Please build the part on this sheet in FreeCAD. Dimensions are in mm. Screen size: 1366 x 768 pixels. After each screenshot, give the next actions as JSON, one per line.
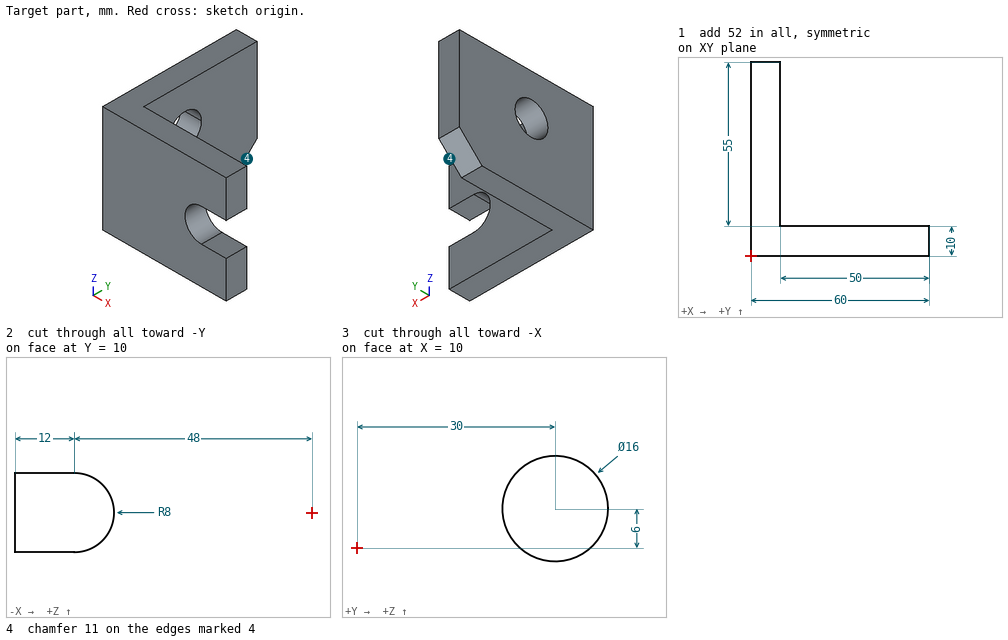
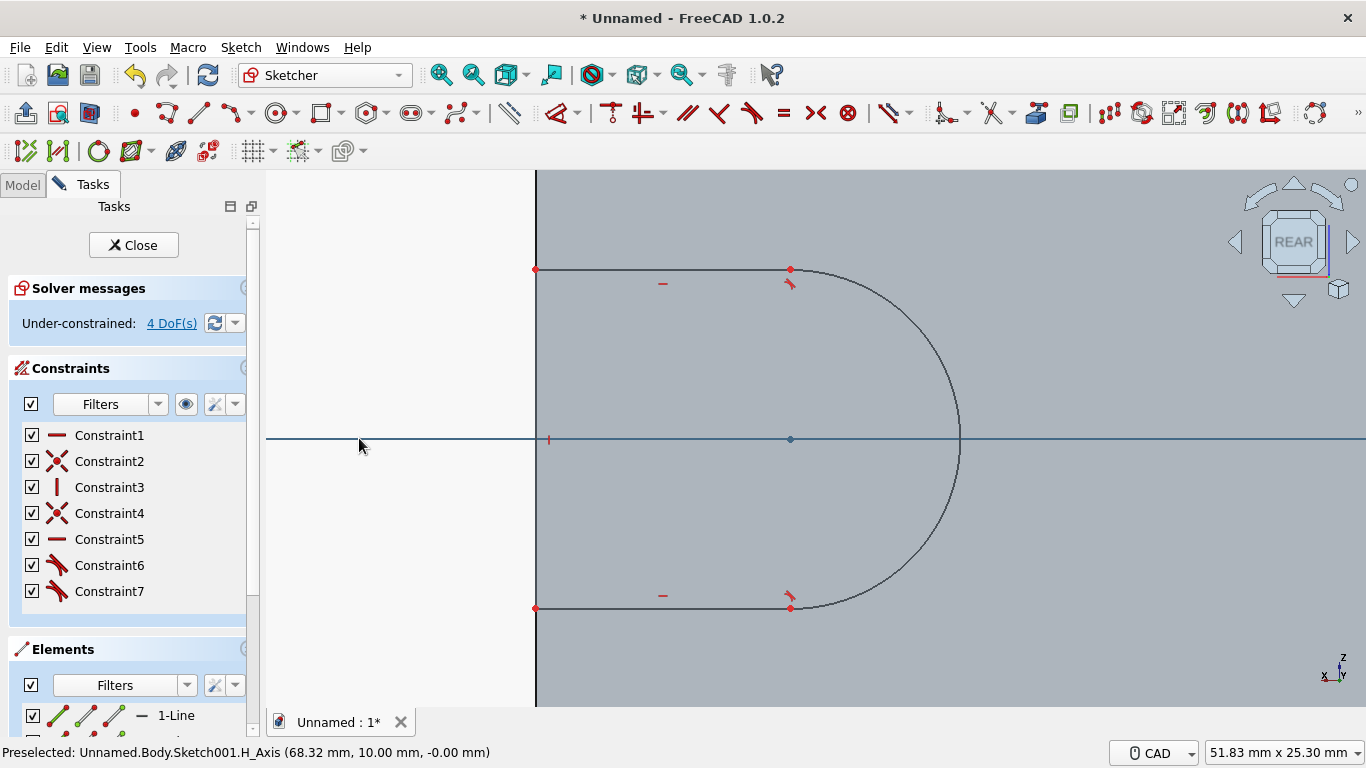
{"action": "left_click", "coordinate": [612, 114]}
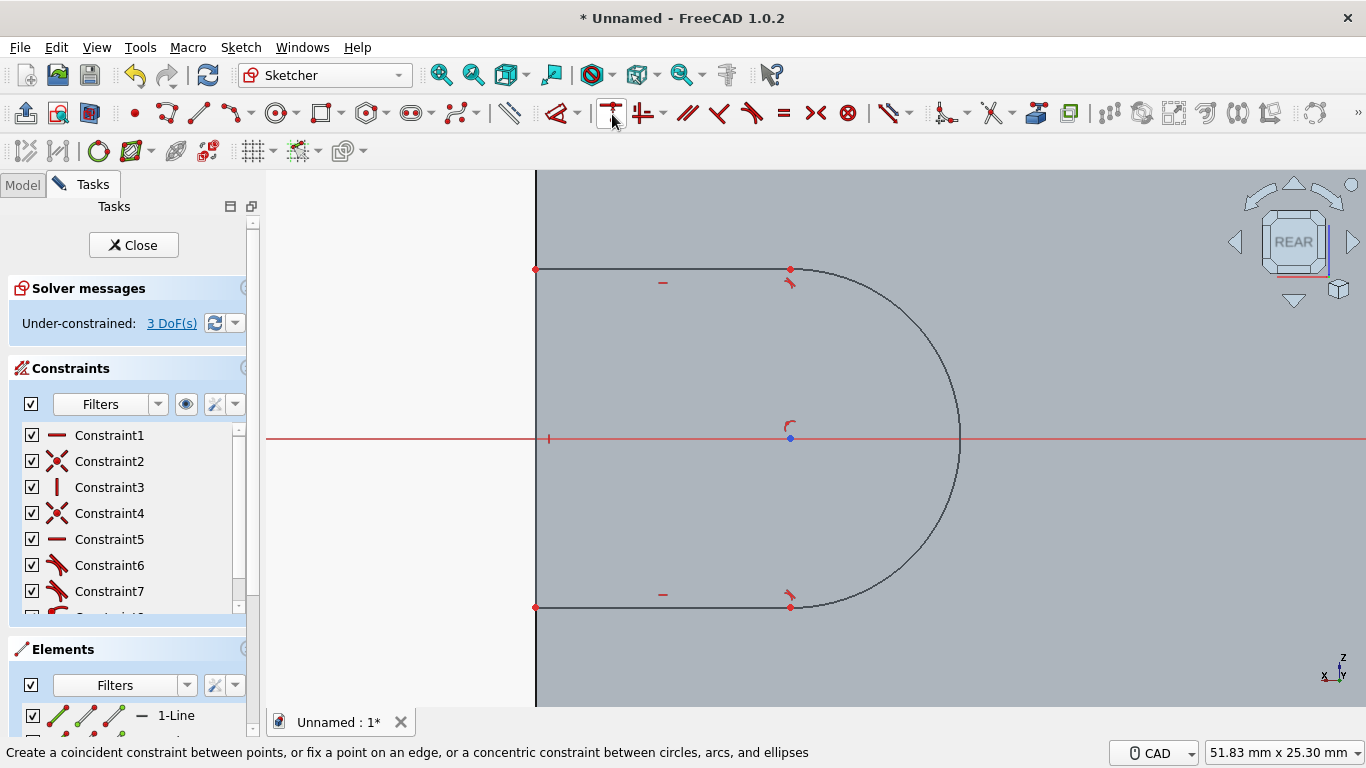
{"action": "left_click", "coordinate": [556, 114]}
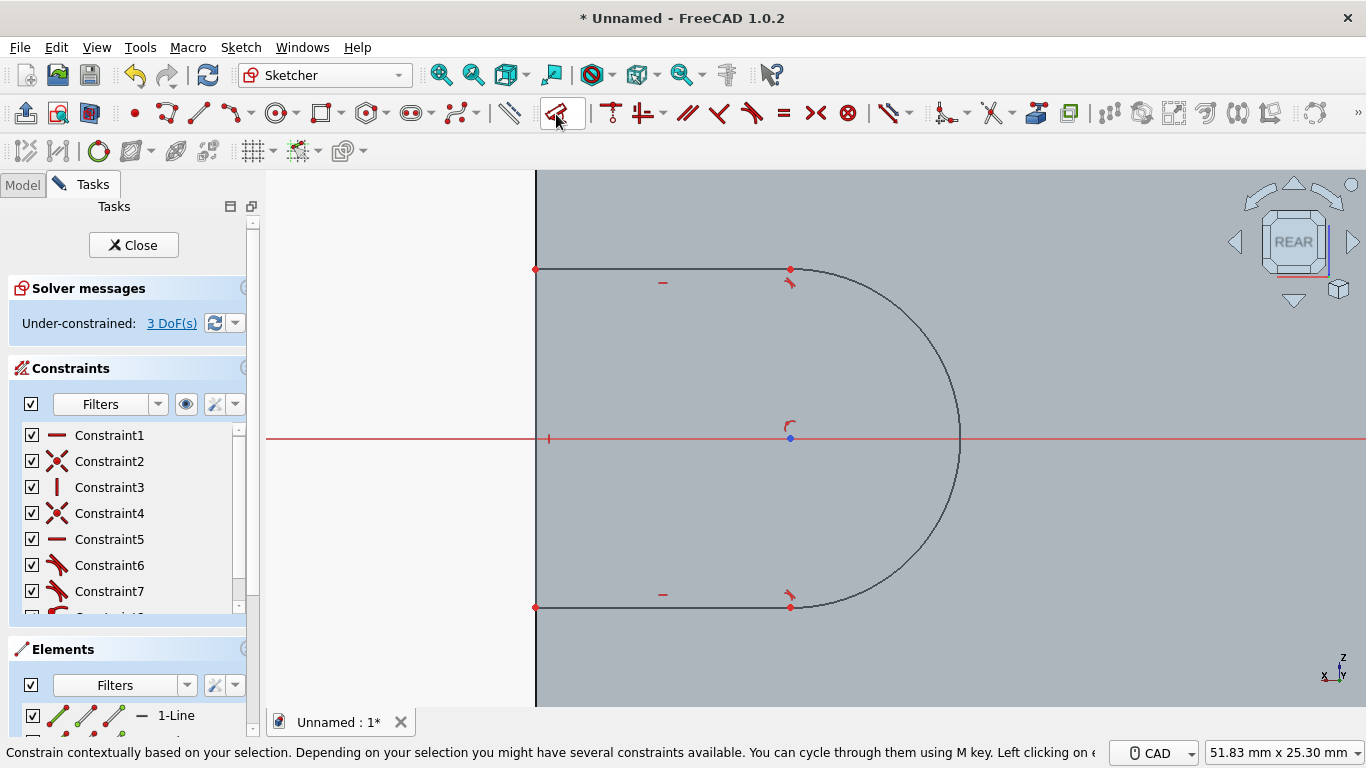
{"action": "left_click", "coordinate": [928, 538]}
{"action": "left_click", "coordinate": [954, 557]}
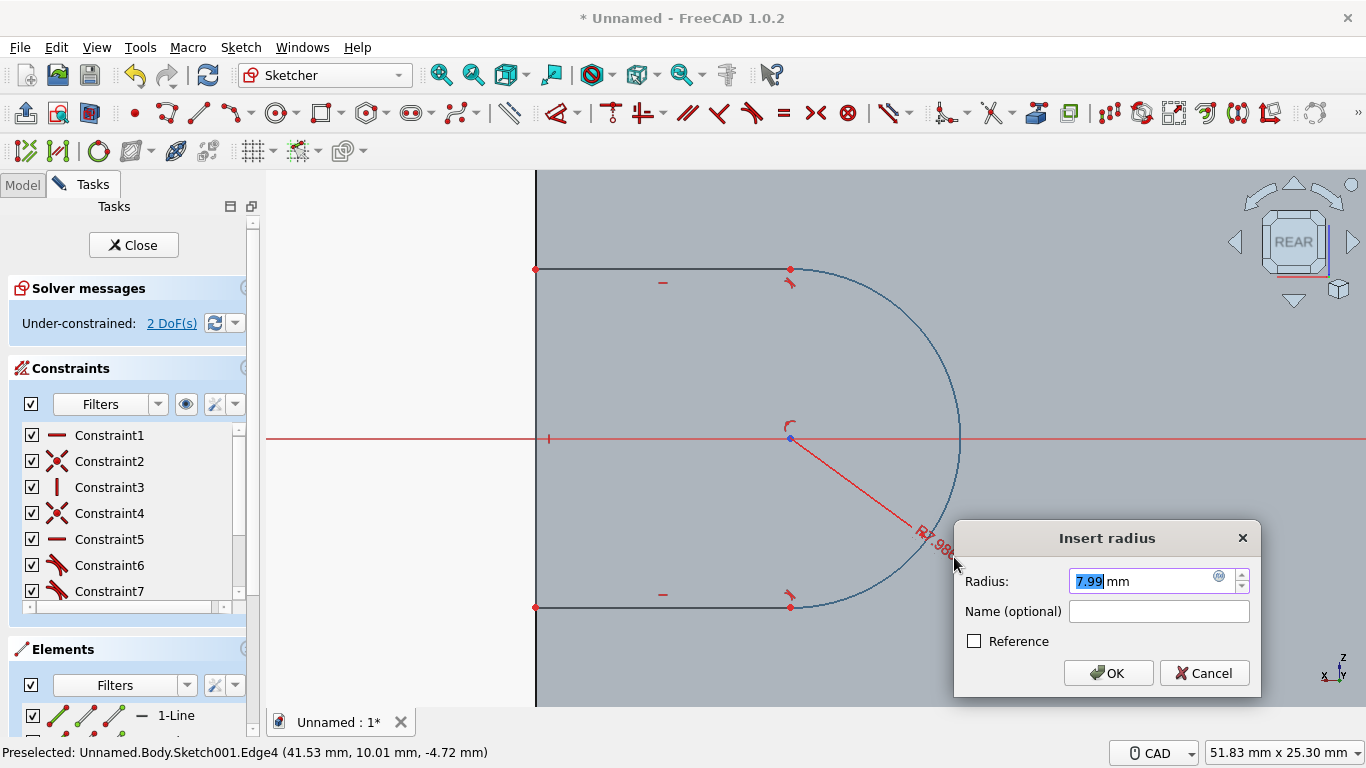
{"action": "type", "text": "8"}
{"action": "key", "text": "Return"}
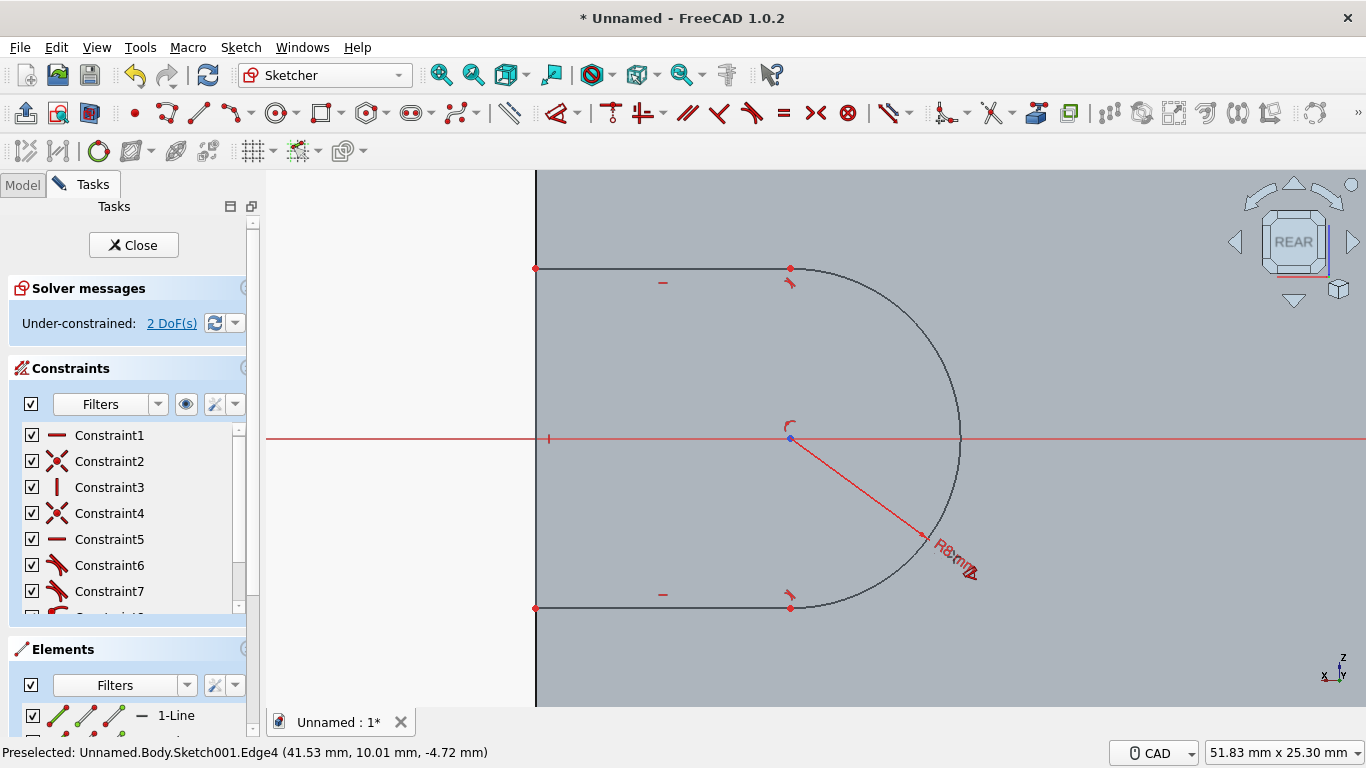
{"action": "left_click", "coordinate": [714, 269]}
{"action": "left_click", "coordinate": [663, 235]}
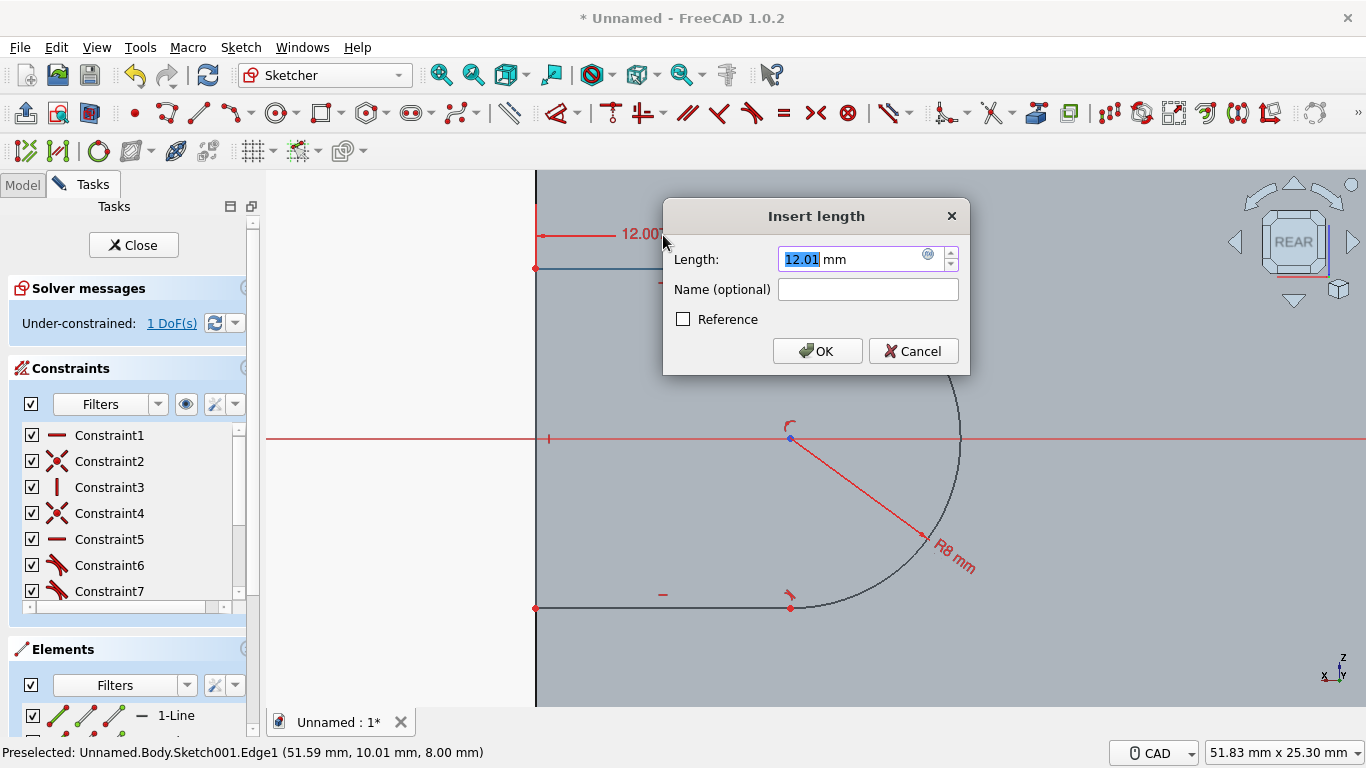
{"action": "type", "text": "12"}
{"action": "key", "text": "Return"}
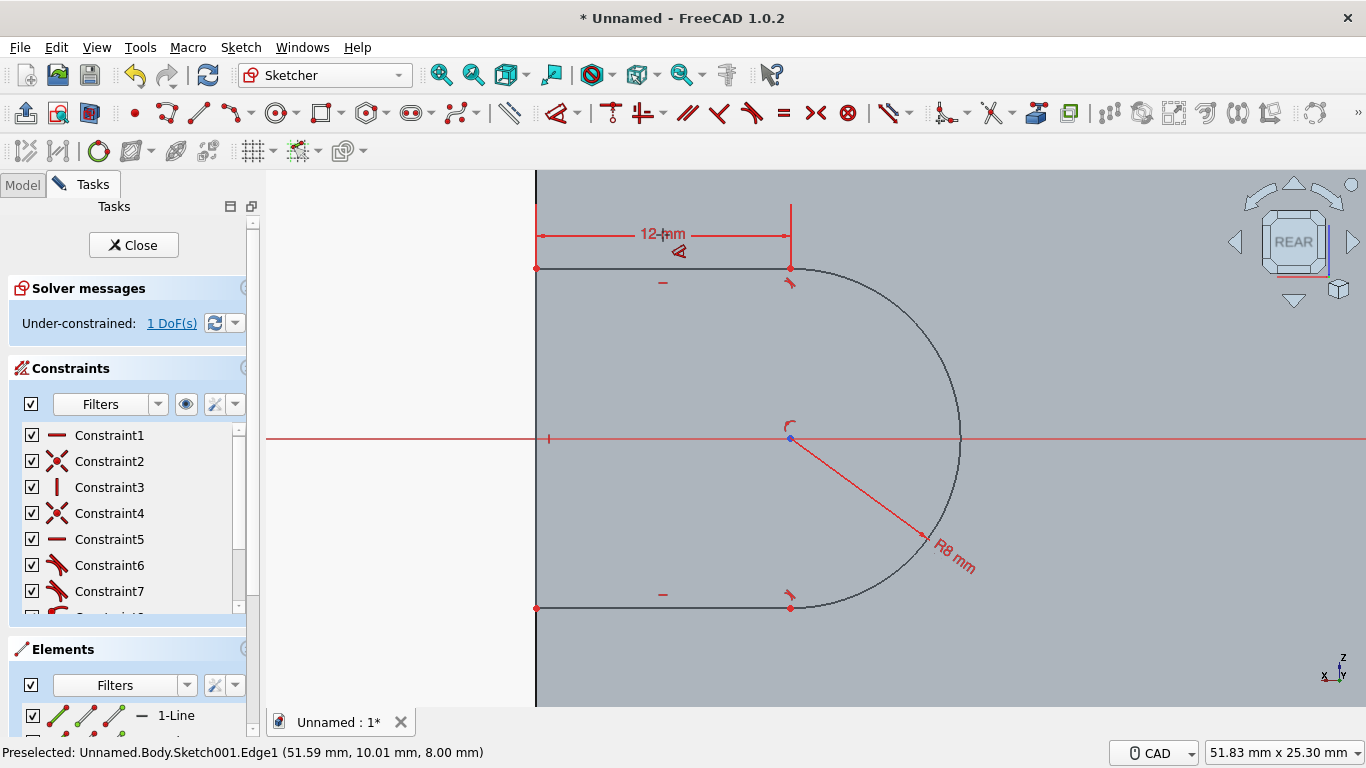
{"action": "left_click", "coordinate": [791, 269]}
{"action": "left_click", "coordinate": [996, 235]}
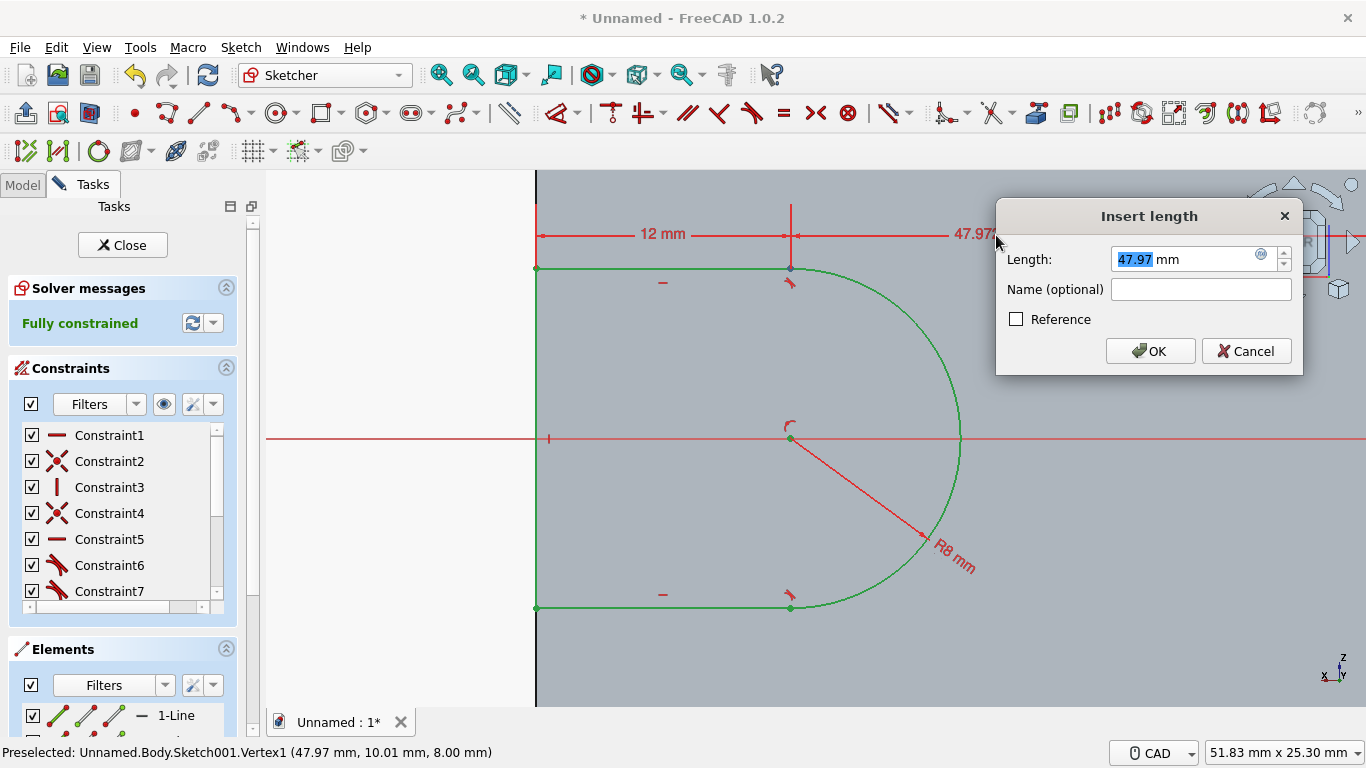
{"action": "type", "text": "48"}
{"action": "key", "text": "Return"}
{"action": "key", "text": "Escape"}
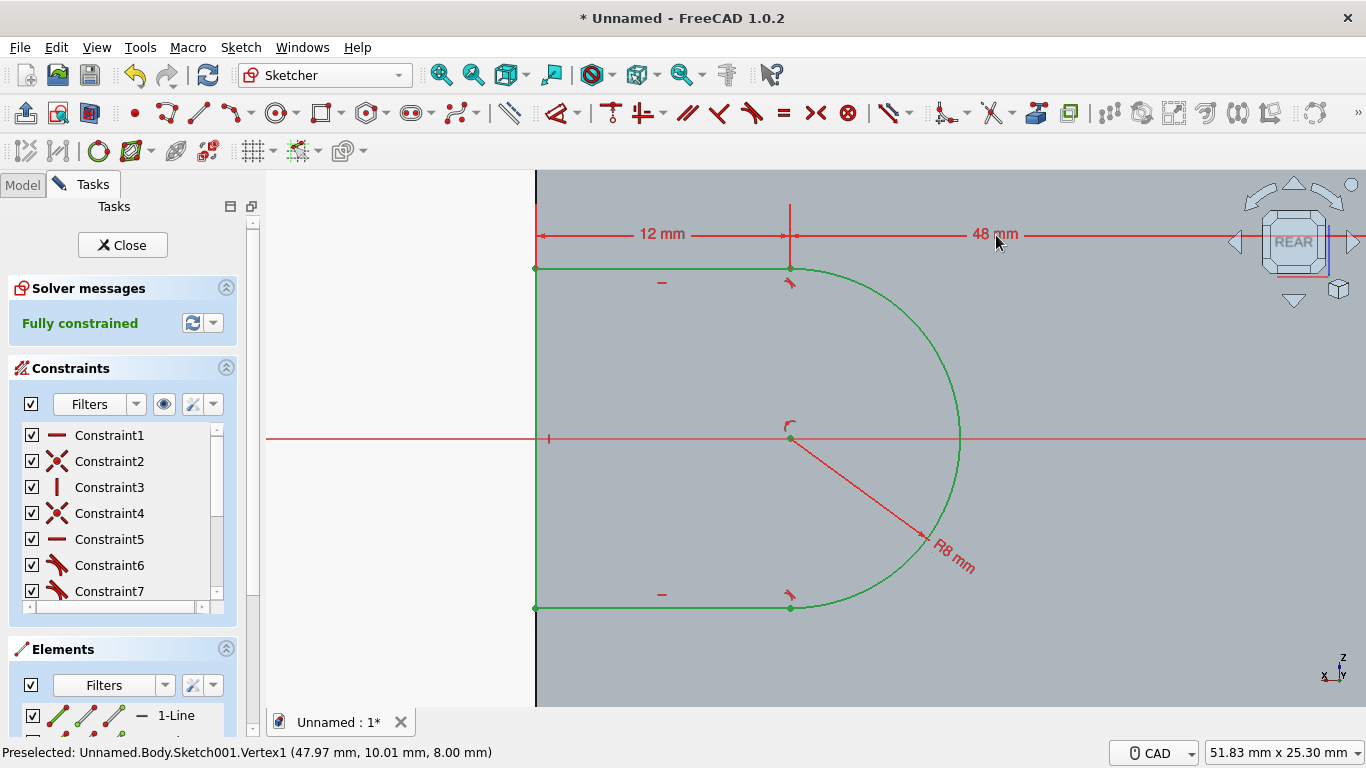
{"action": "left_click", "coordinate": [123, 245]}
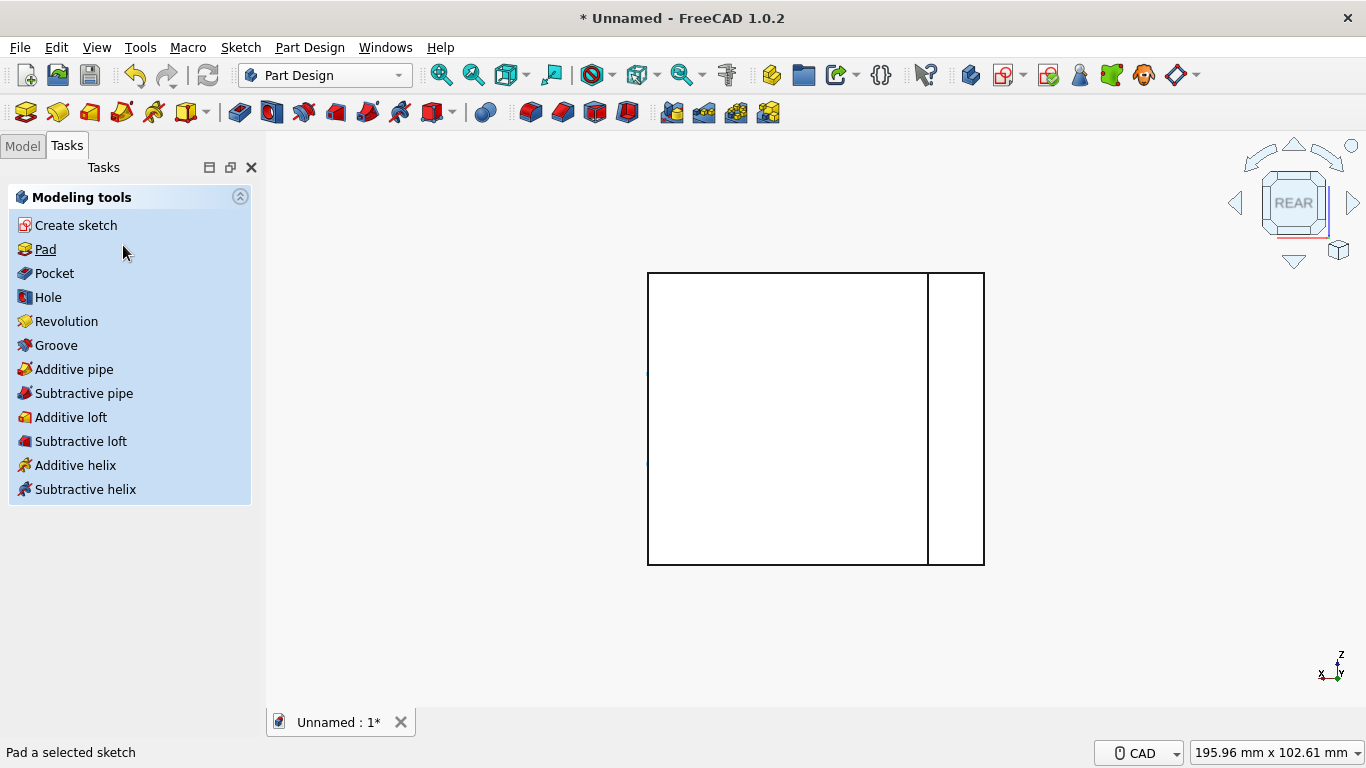
{"action": "left_click", "coordinate": [240, 112]}